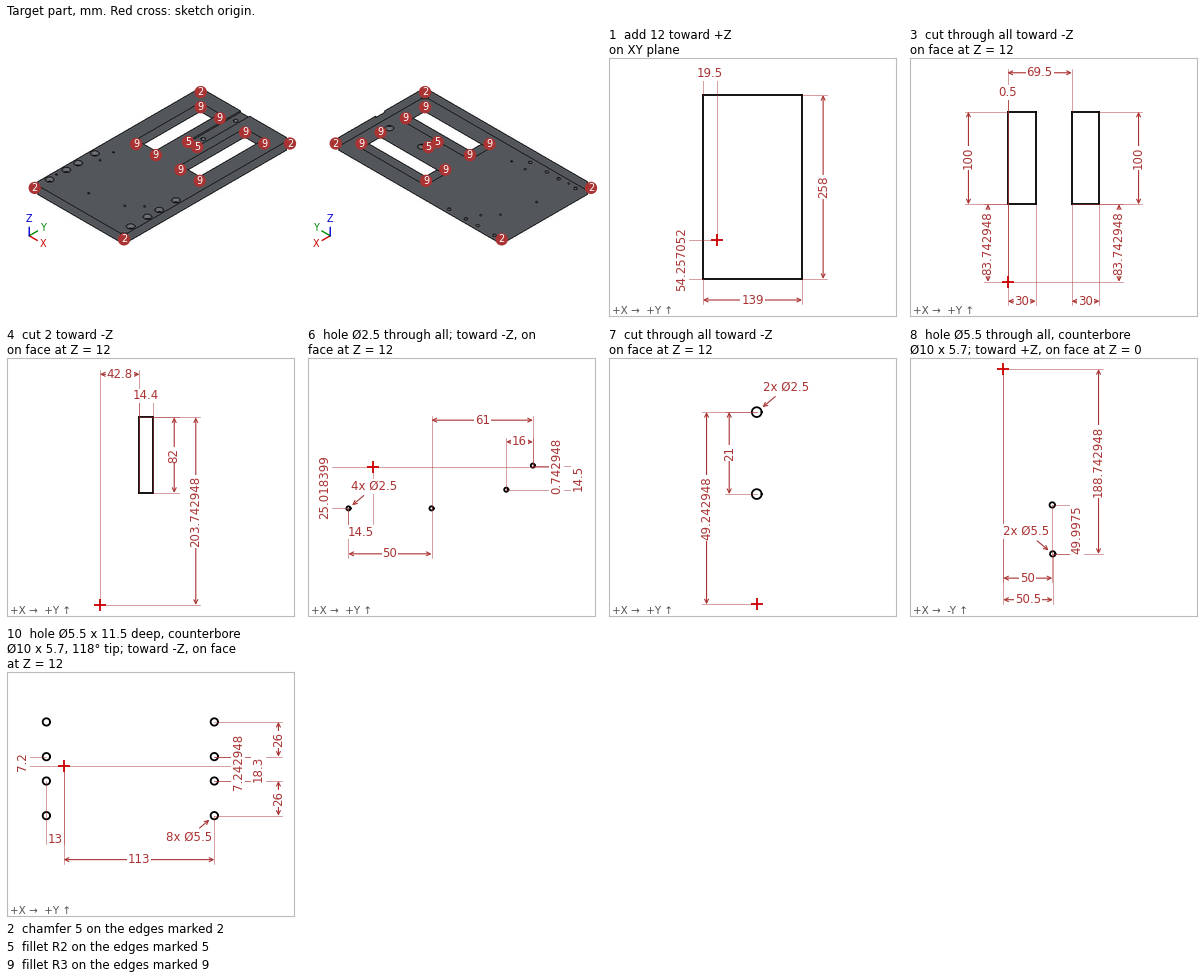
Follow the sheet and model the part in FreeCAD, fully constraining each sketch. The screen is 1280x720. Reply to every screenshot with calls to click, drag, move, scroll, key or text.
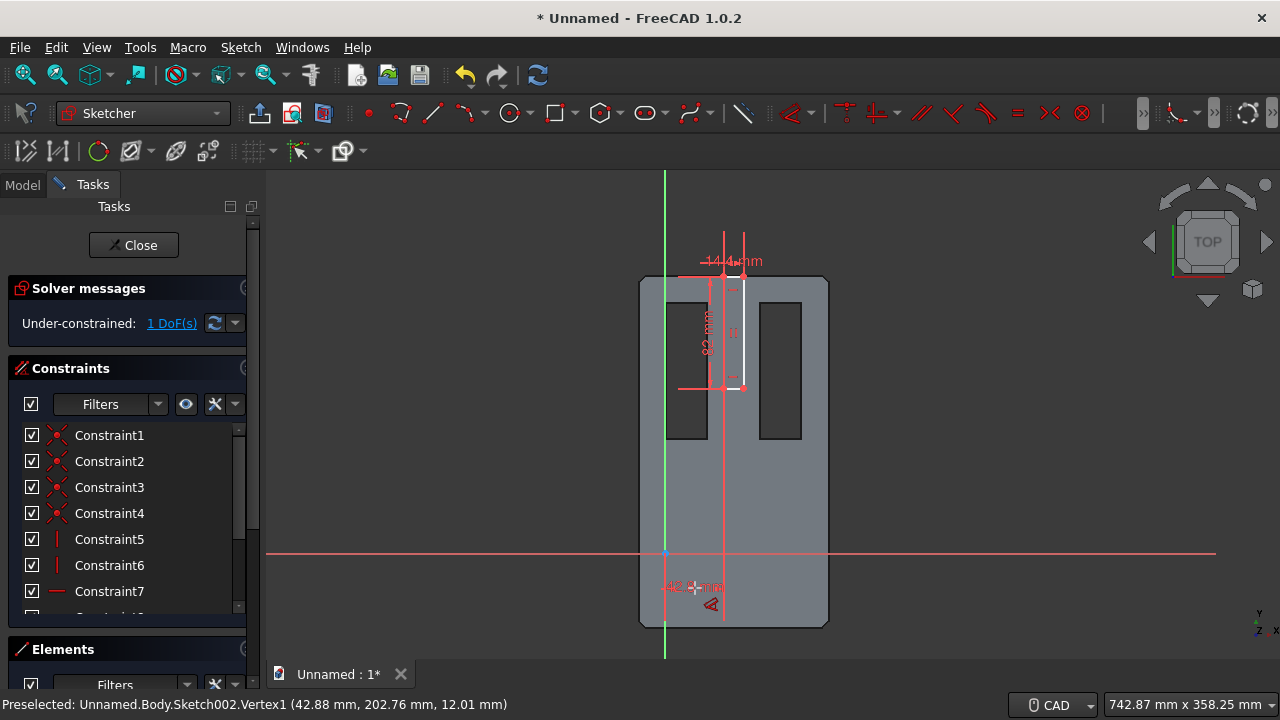
click(724, 277)
click(631, 415)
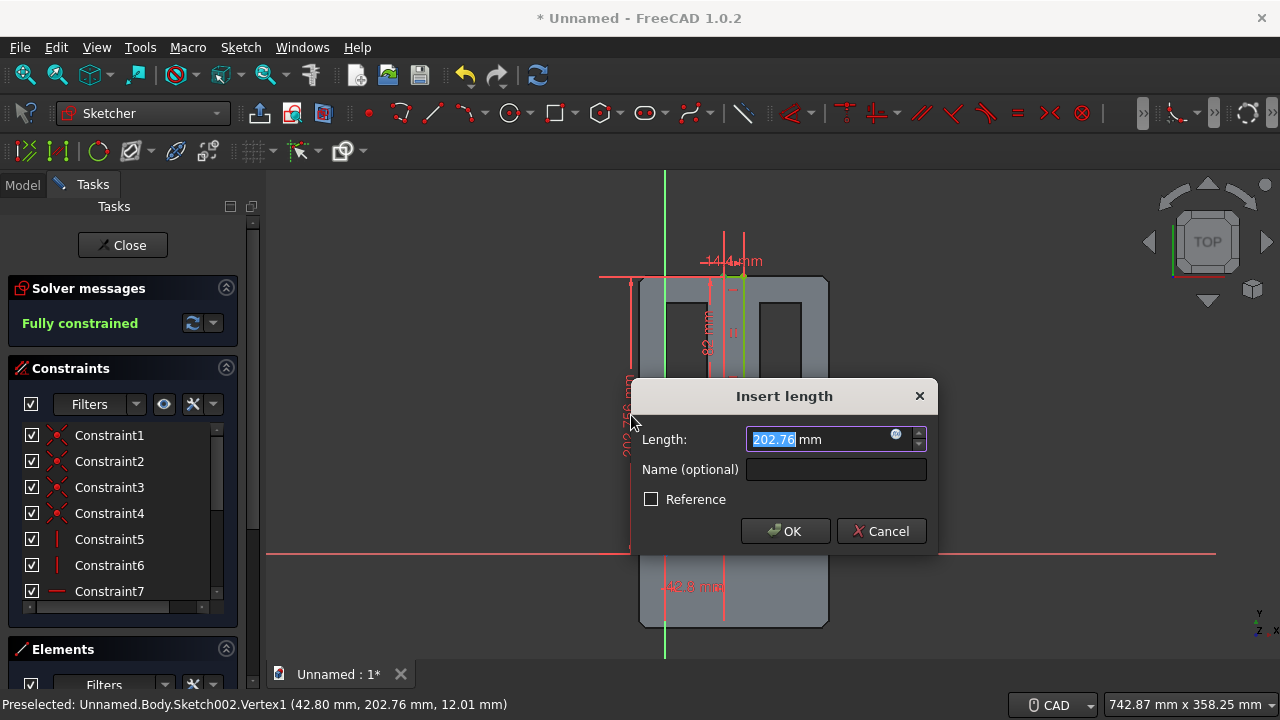
text(203.742948)
key(Return)
key(Escape)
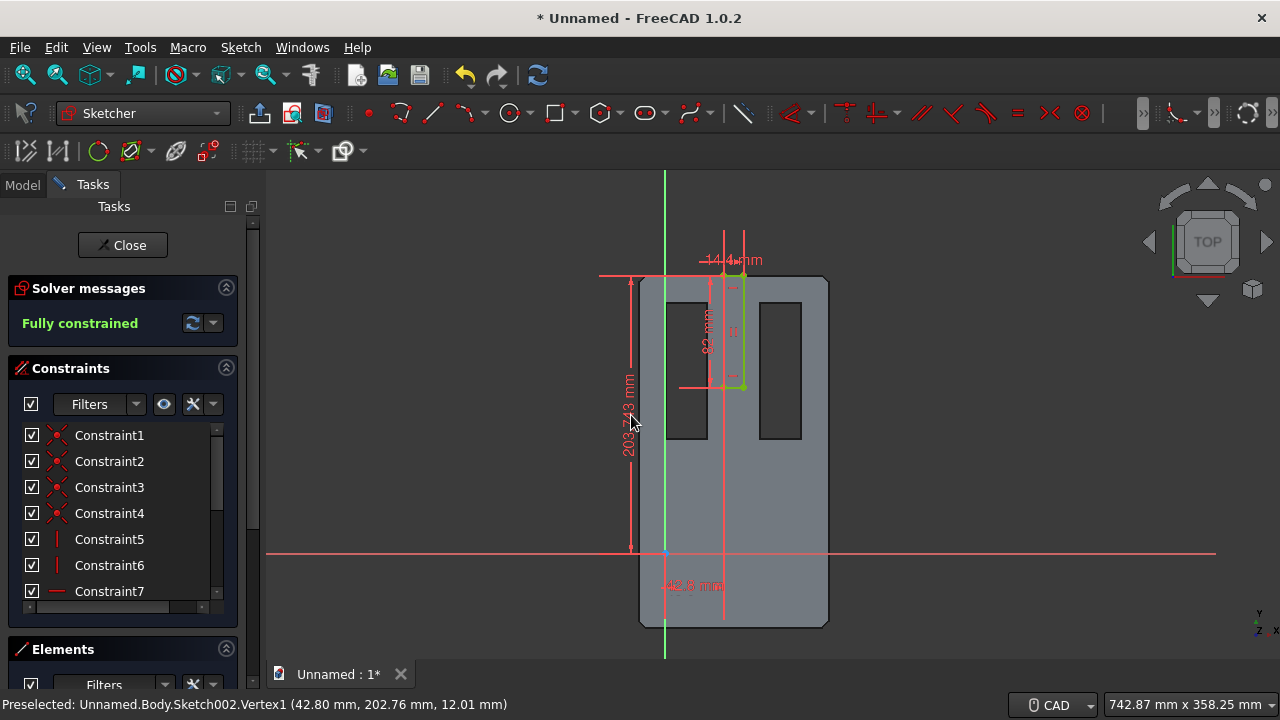
click(123, 245)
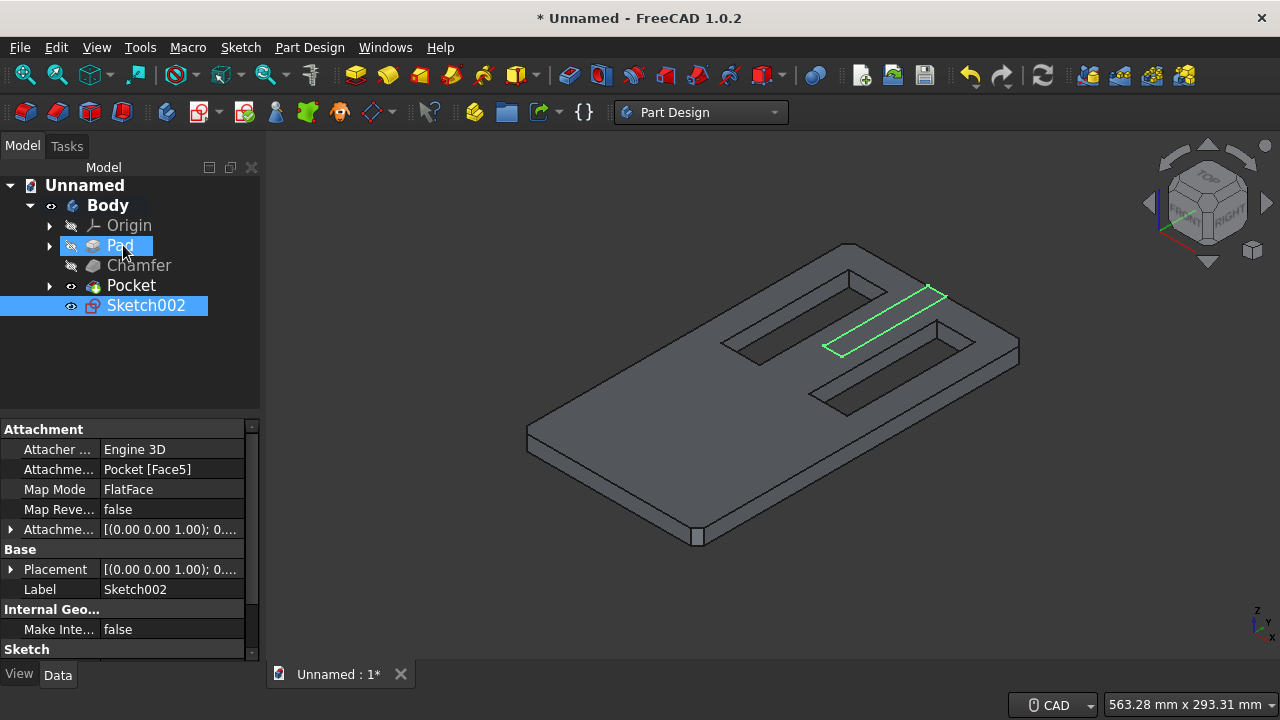
click(570, 76)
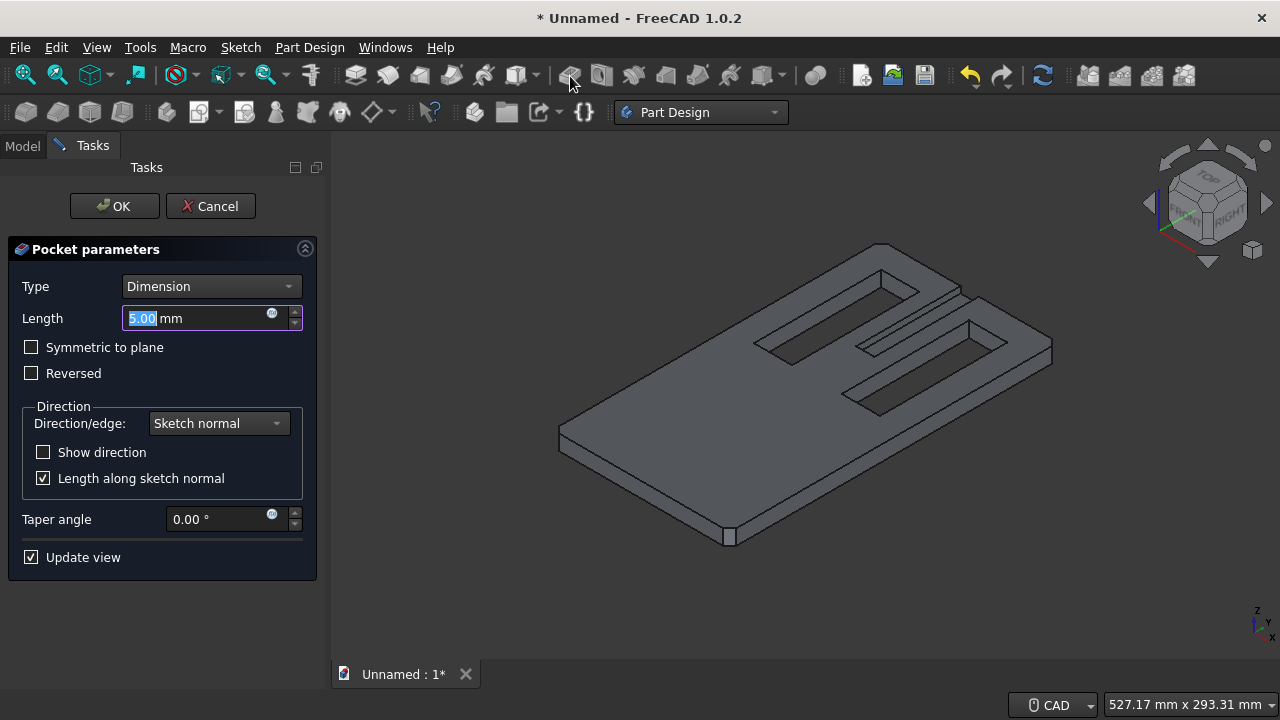
text(2)
key(Tab)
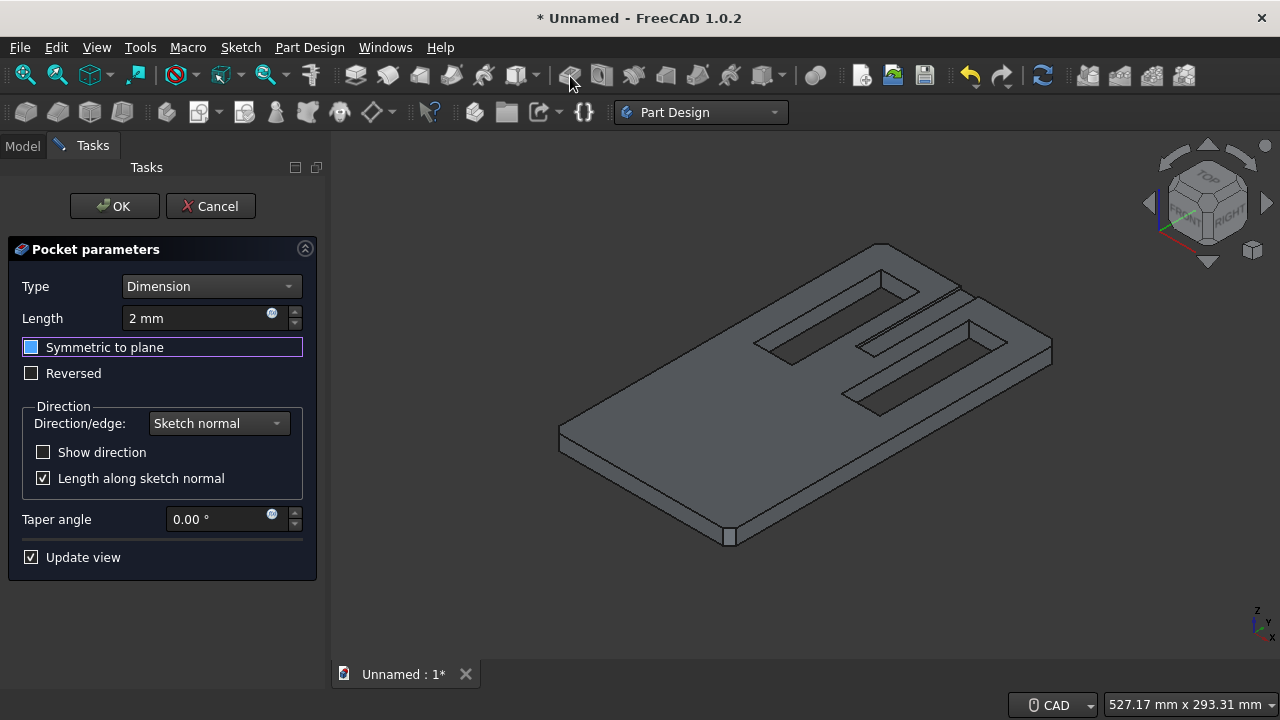
click(115, 206)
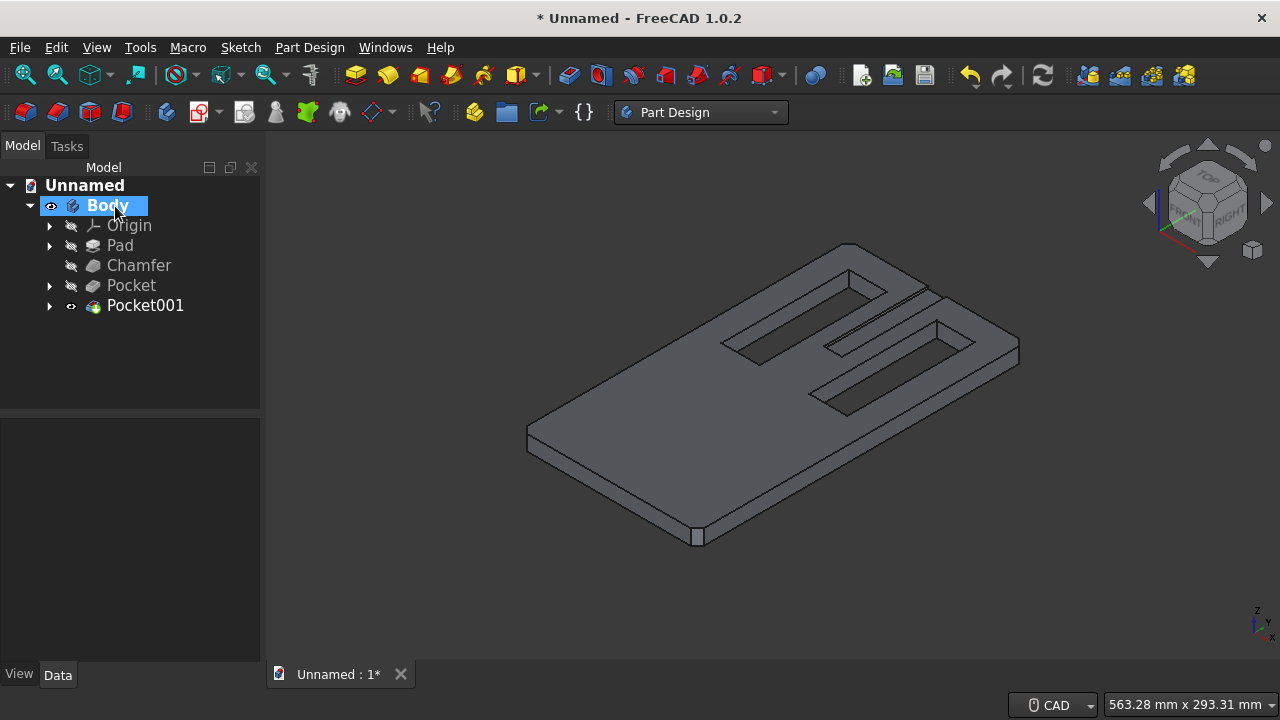
scroll(842, 357, up, 13)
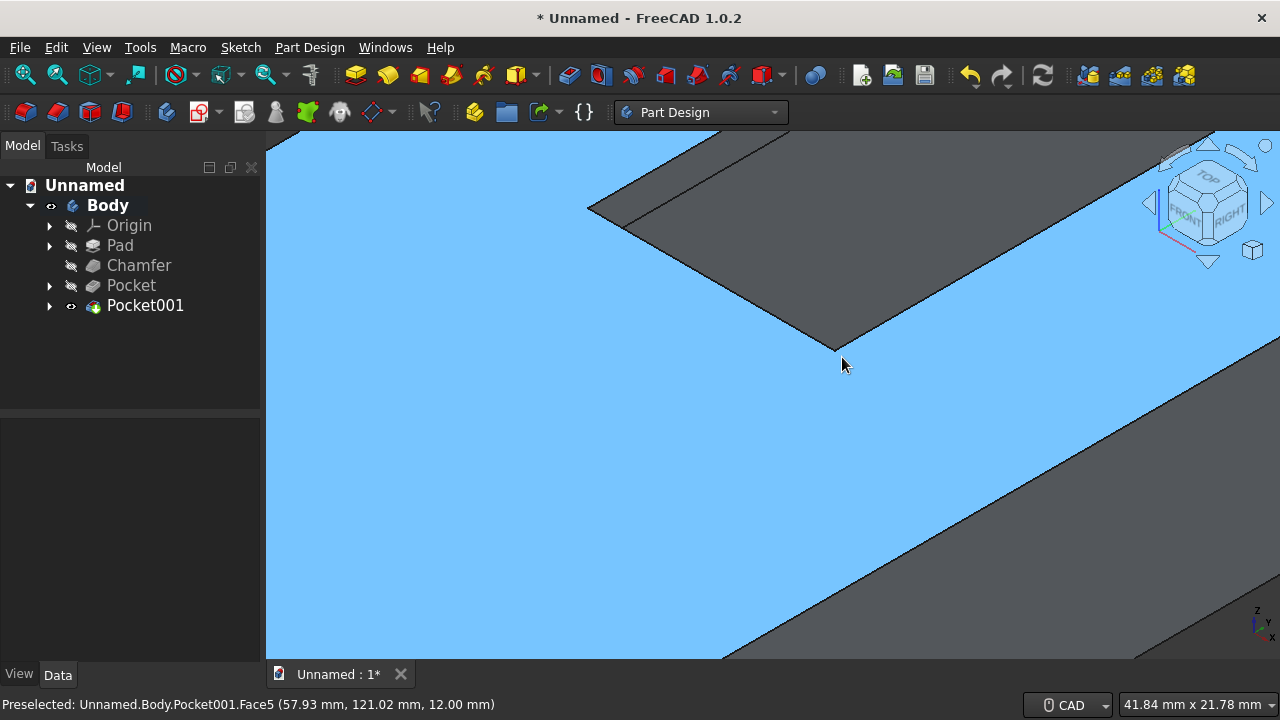
key(v)
key(f)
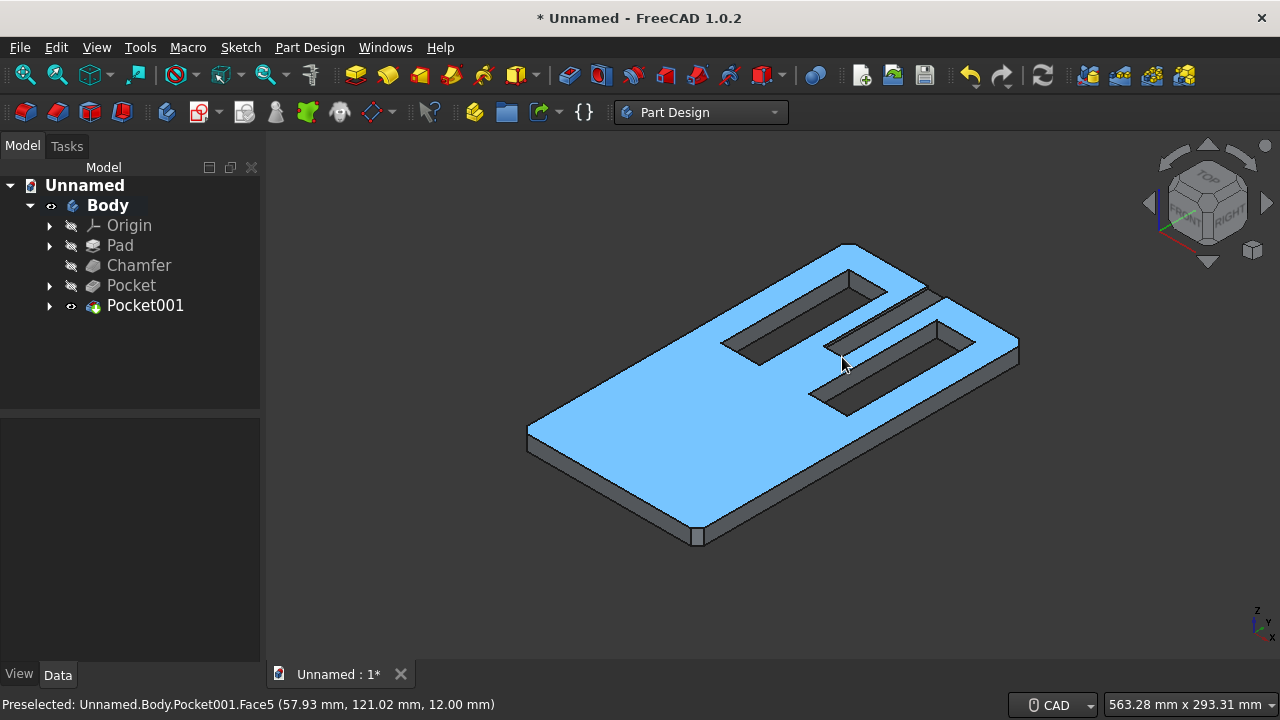
key(2)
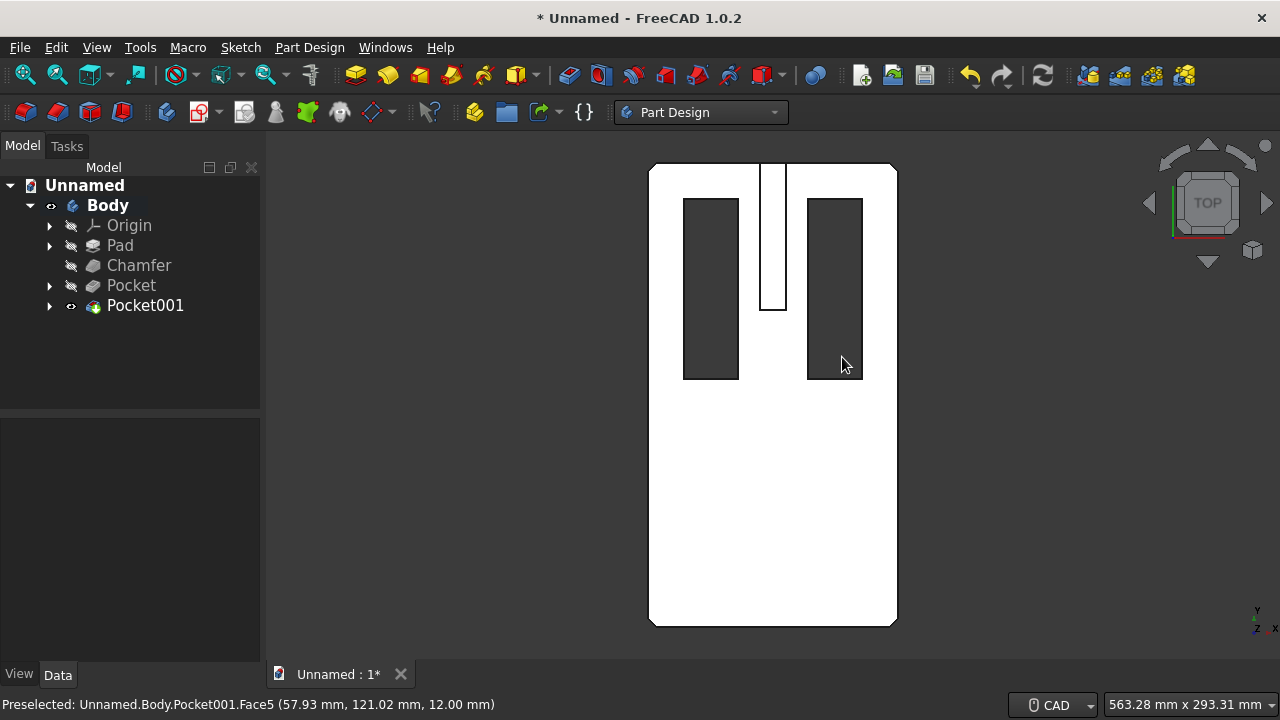
scroll(786, 309, up, 13)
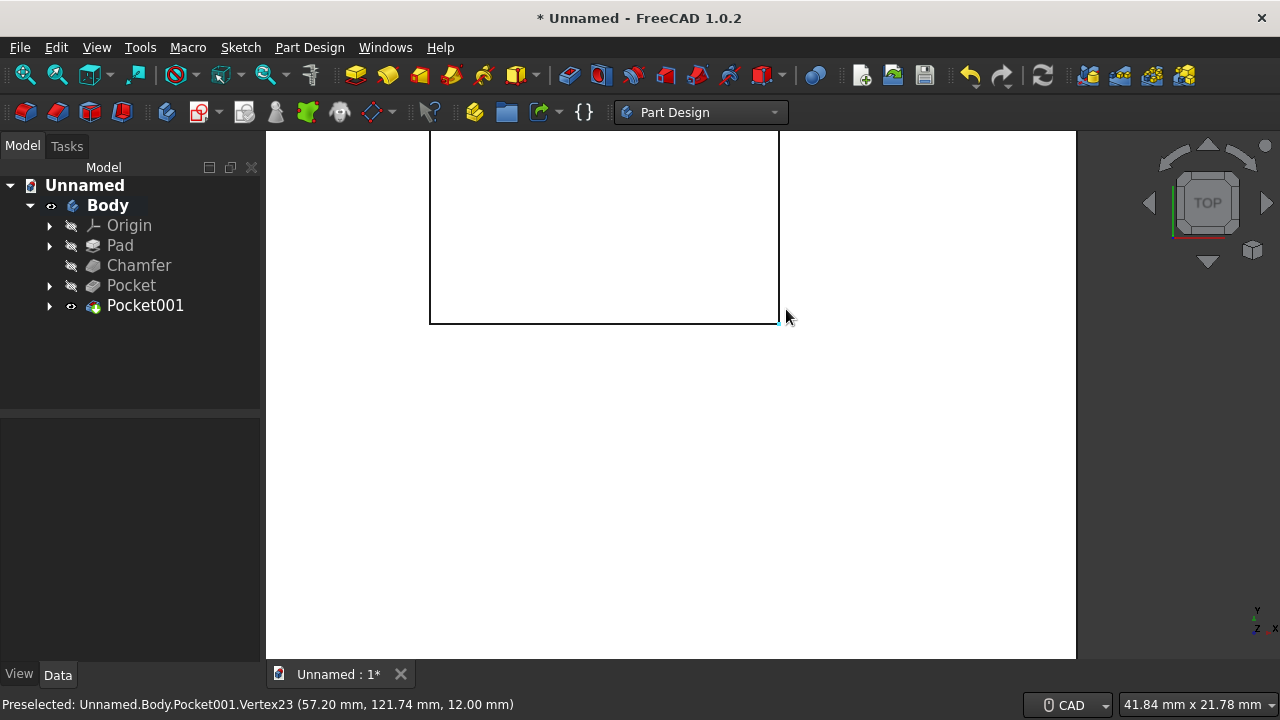
click(26, 76)